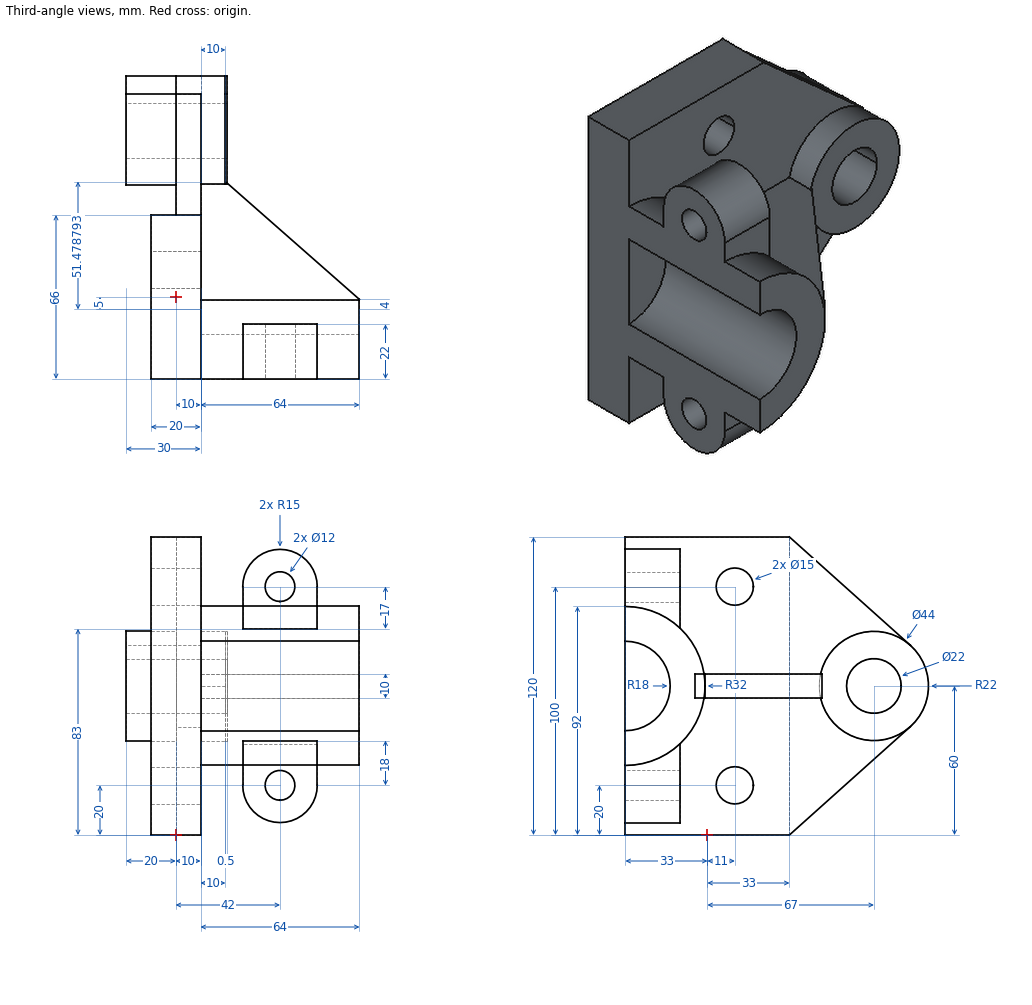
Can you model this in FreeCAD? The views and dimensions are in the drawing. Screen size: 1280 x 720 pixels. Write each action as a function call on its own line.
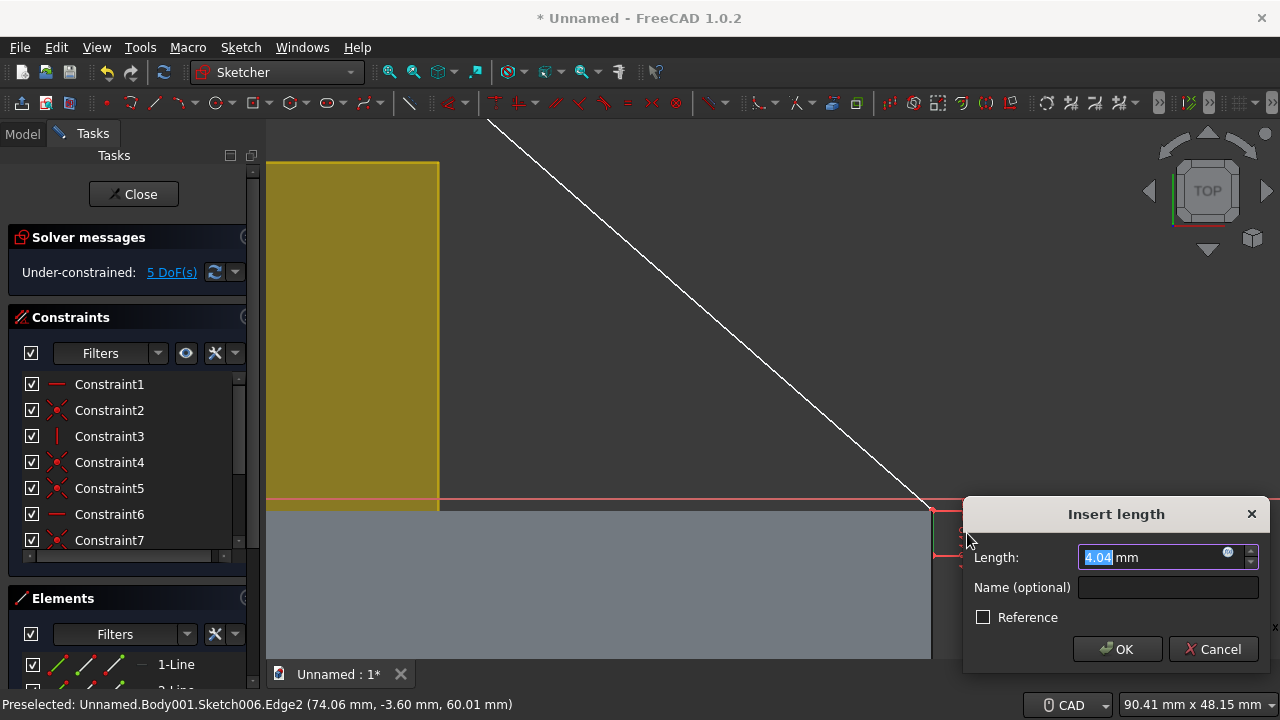
text(4)
key(Return)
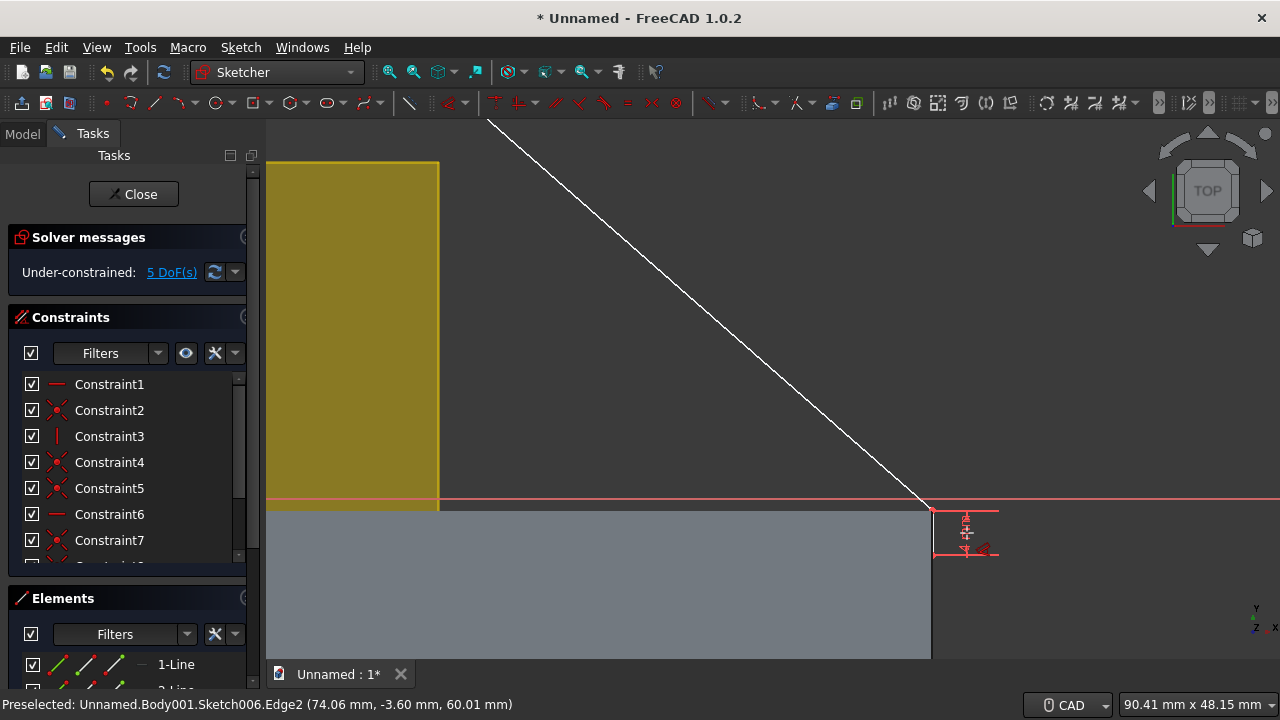
click(430, 555)
click(613, 589)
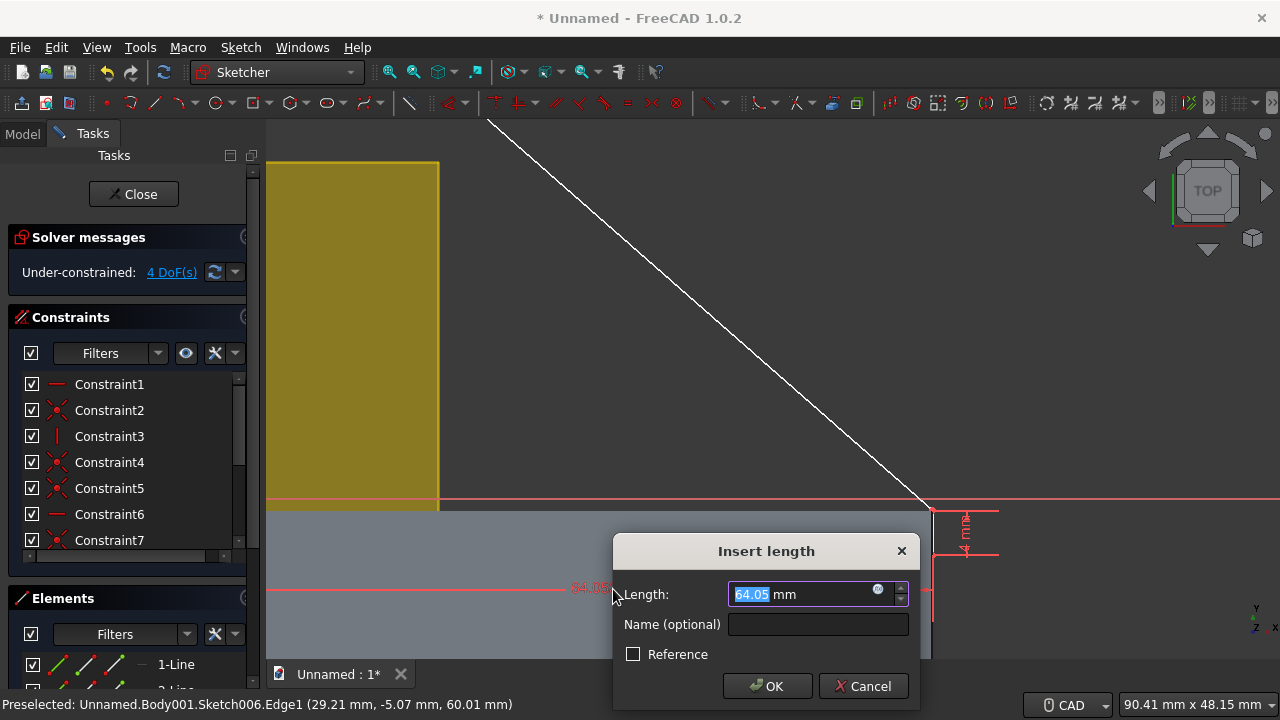
text(64)
key(Return)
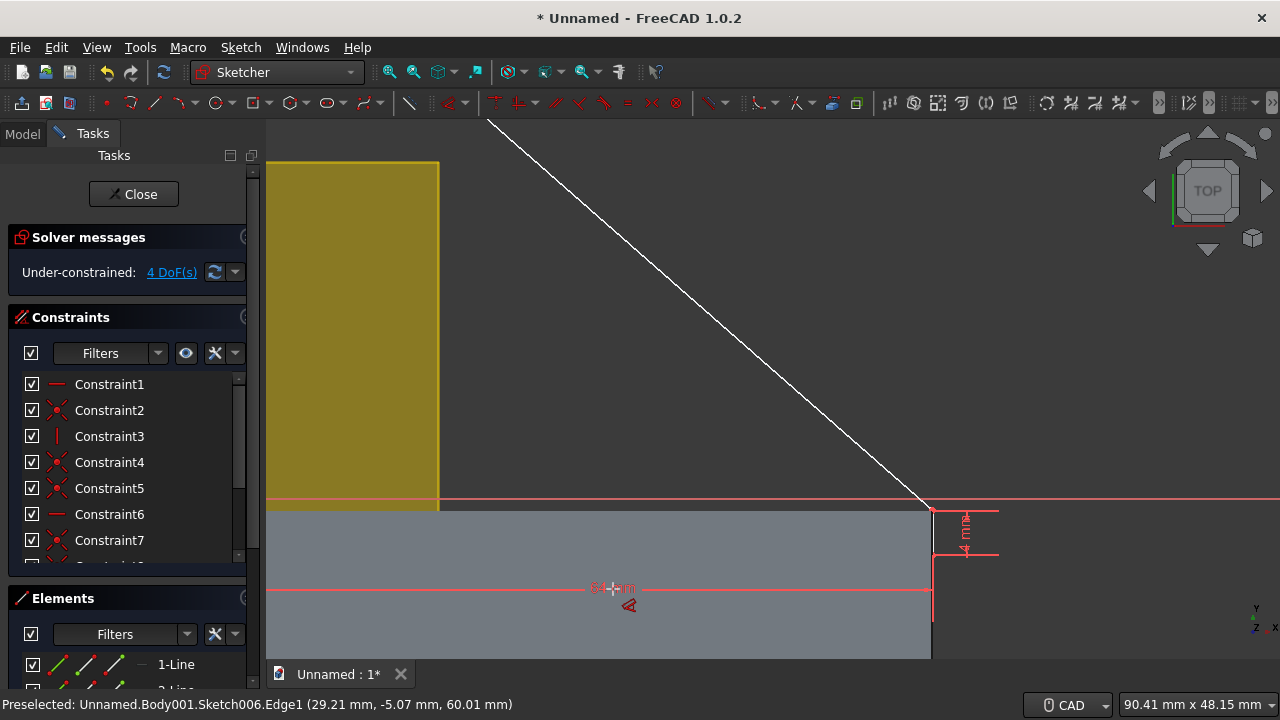
scroll(932, 539, down, 3)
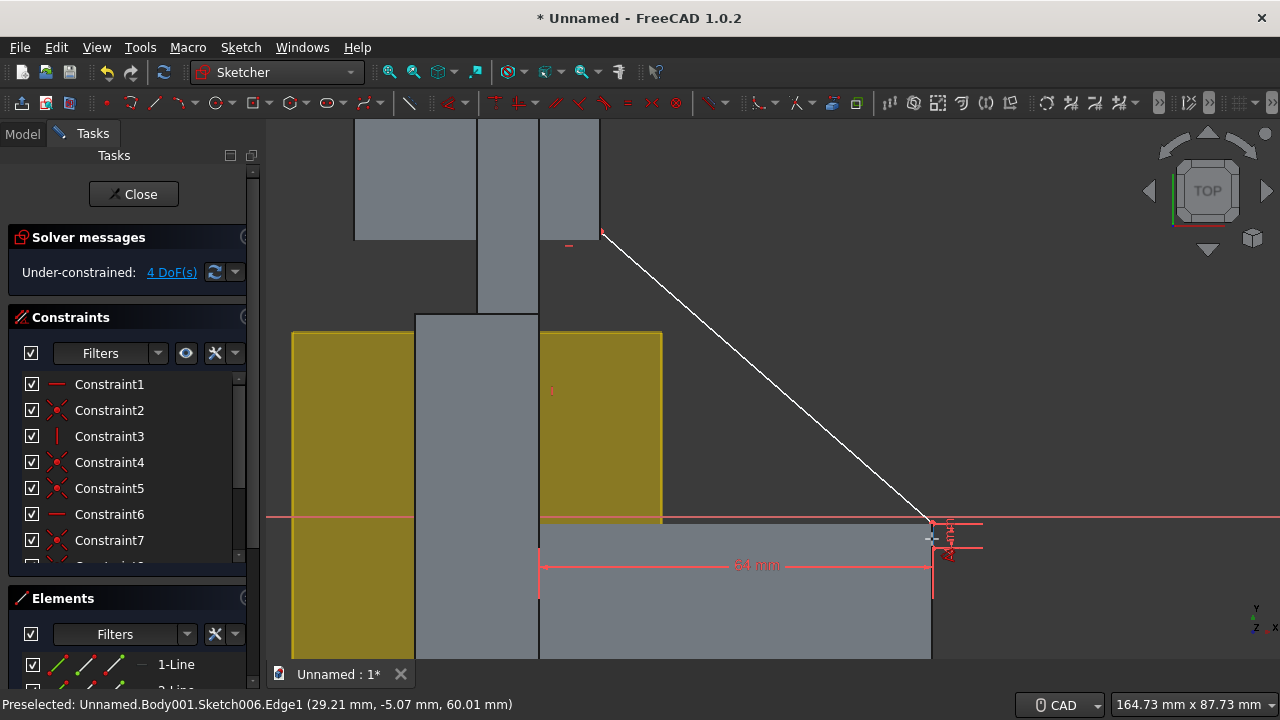
click(582, 232)
click(570, 198)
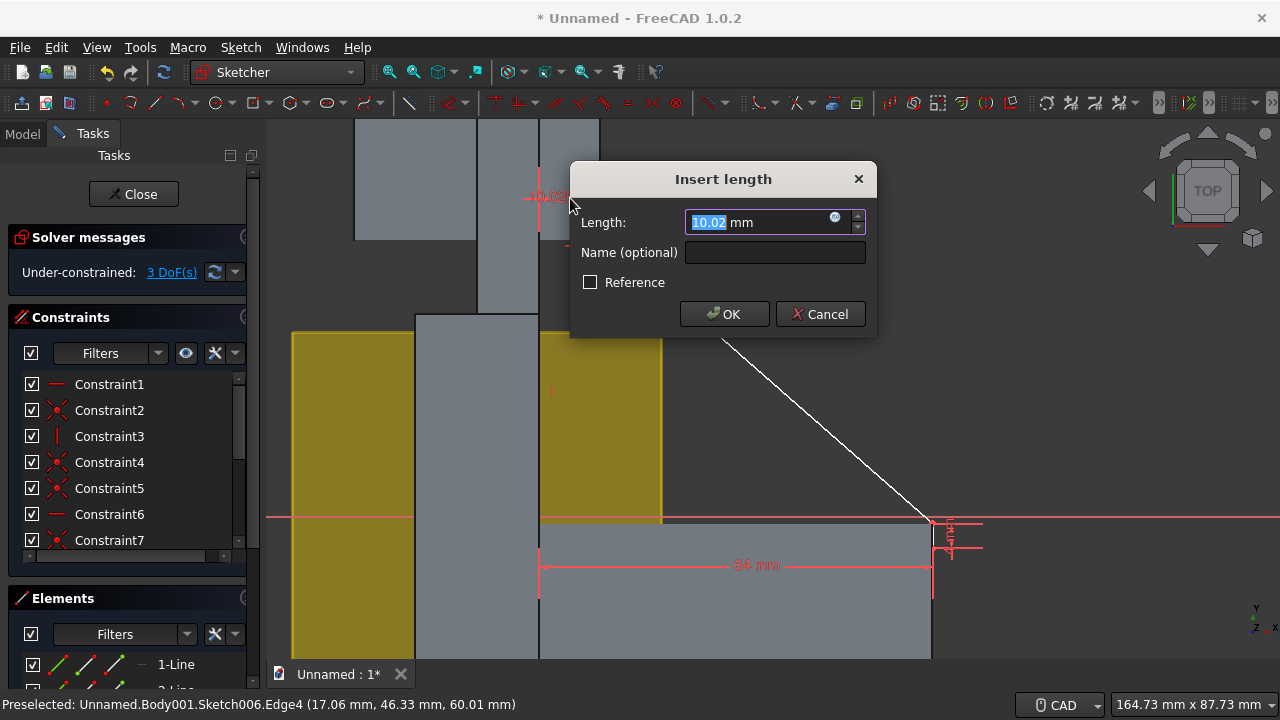
text(10)
key(Return)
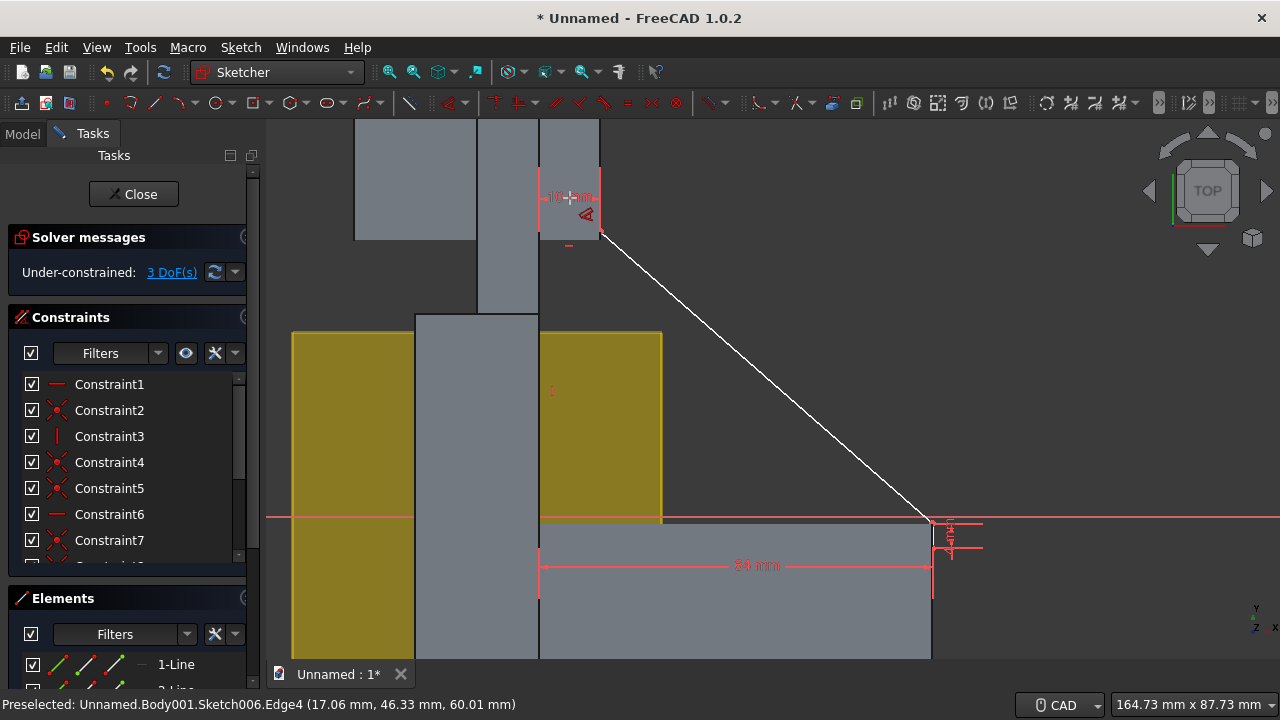
scroll(539, 548, up, 2)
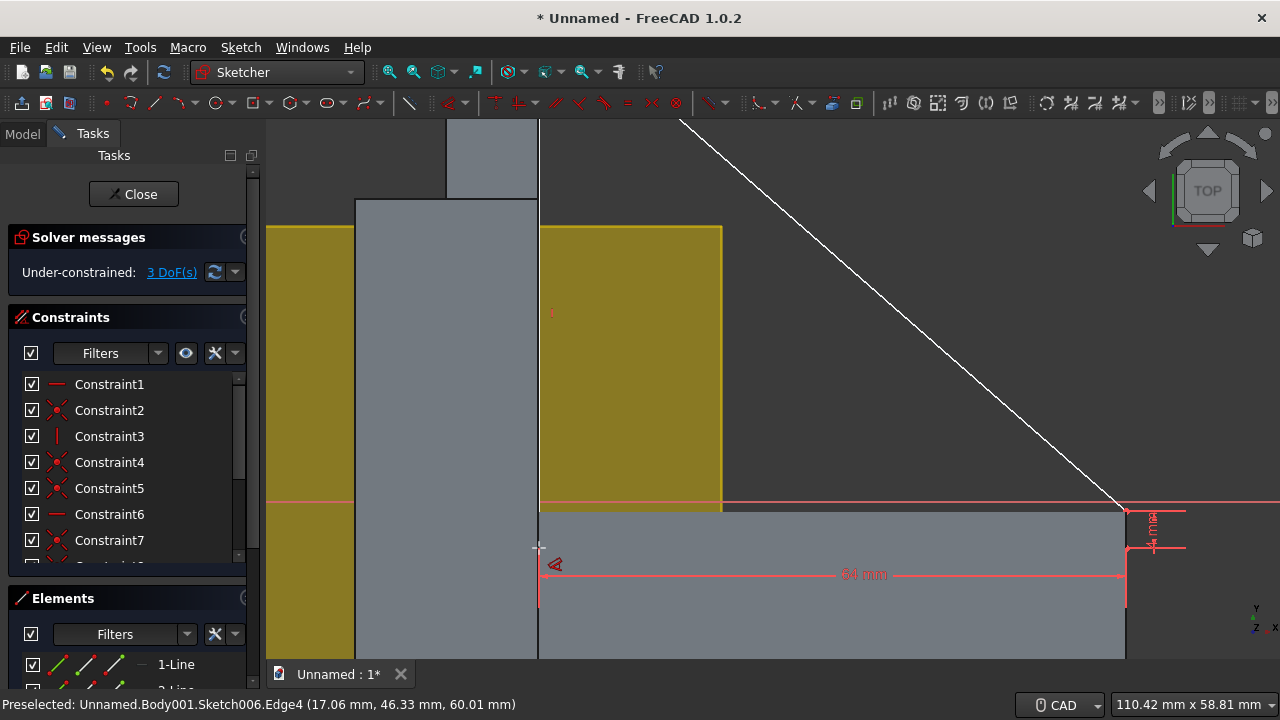
click(539, 548)
click(412, 525)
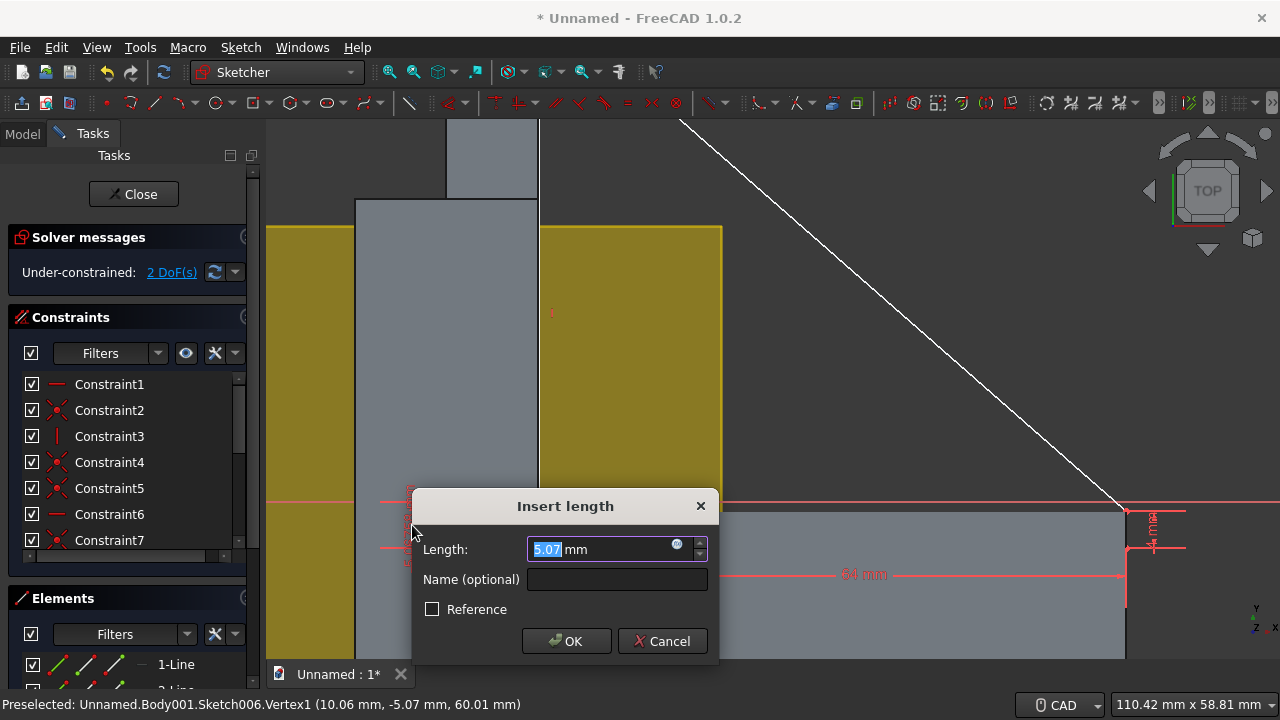
text(5)
key(Return)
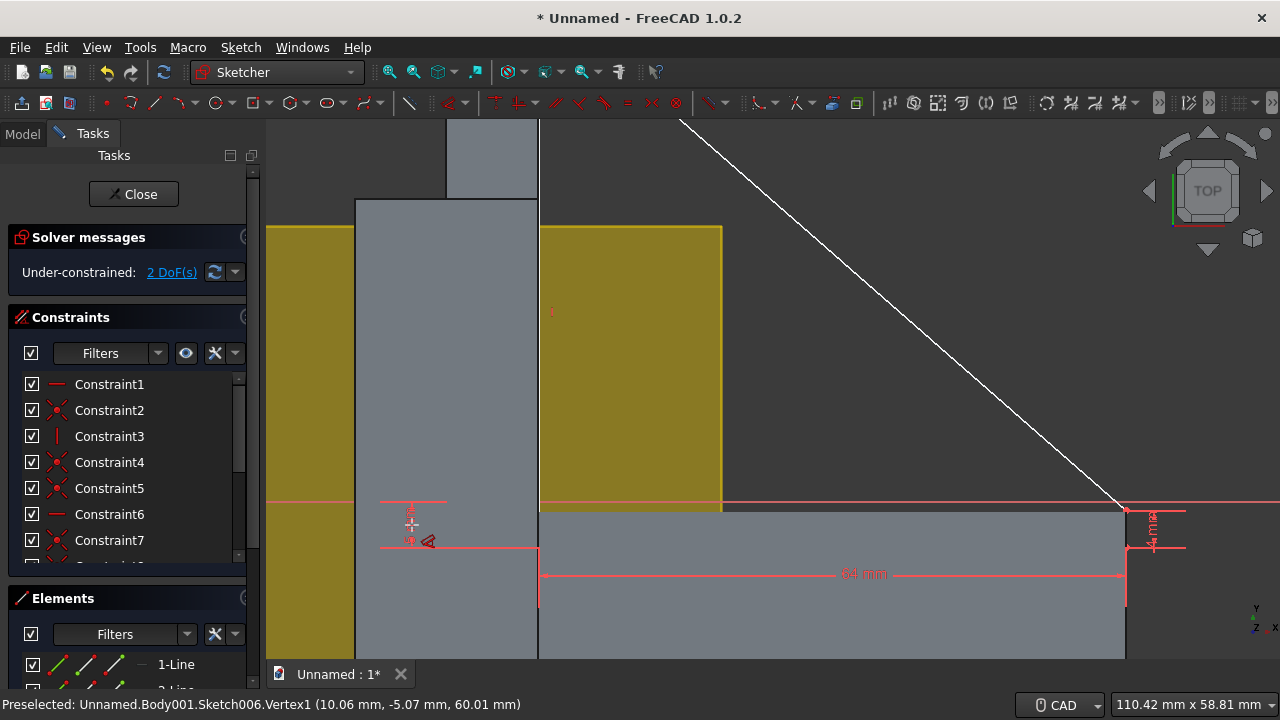
click(539, 548)
click(493, 582)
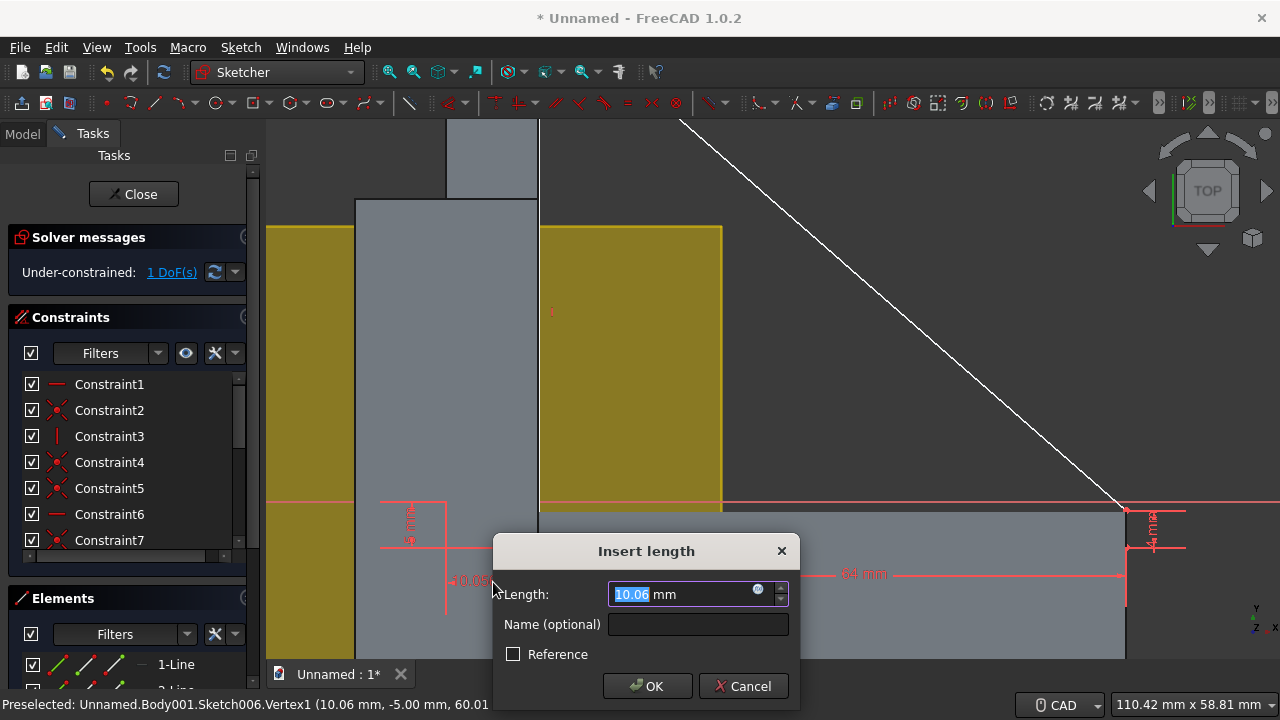
text(10)
key(Return)